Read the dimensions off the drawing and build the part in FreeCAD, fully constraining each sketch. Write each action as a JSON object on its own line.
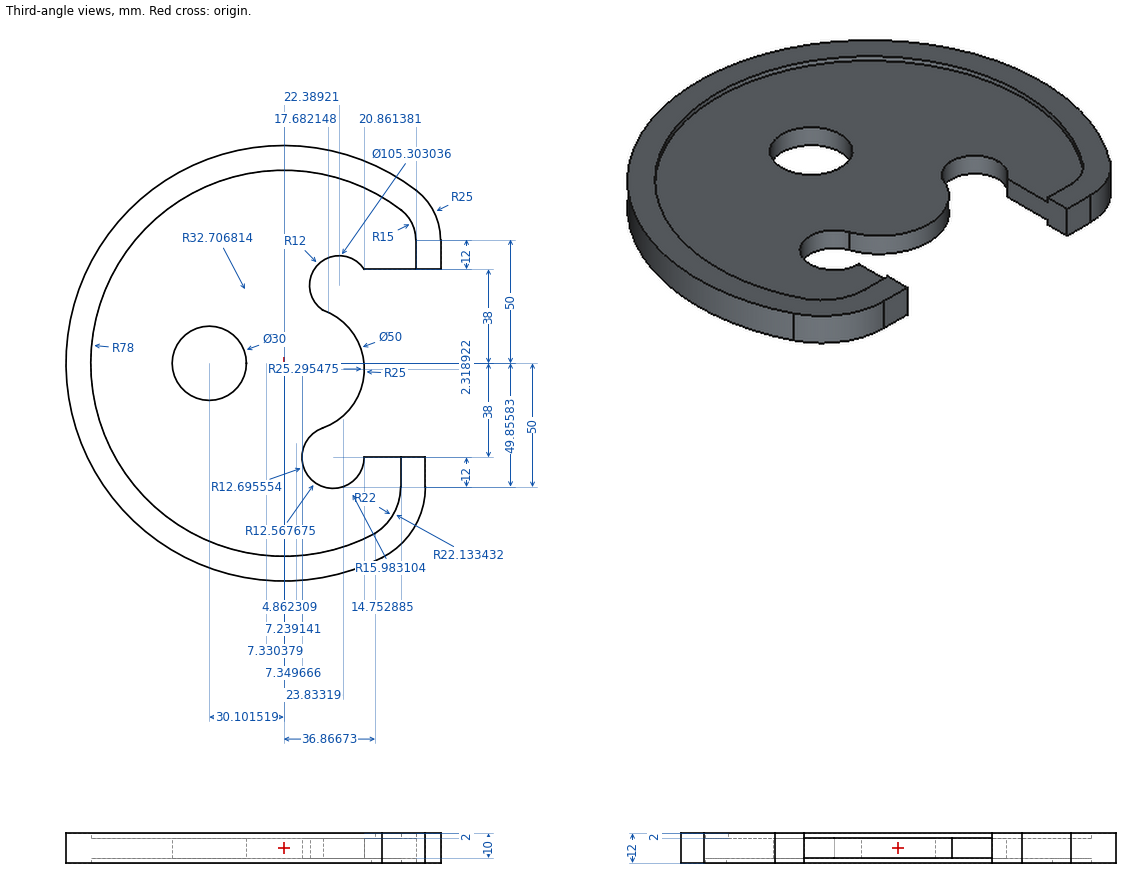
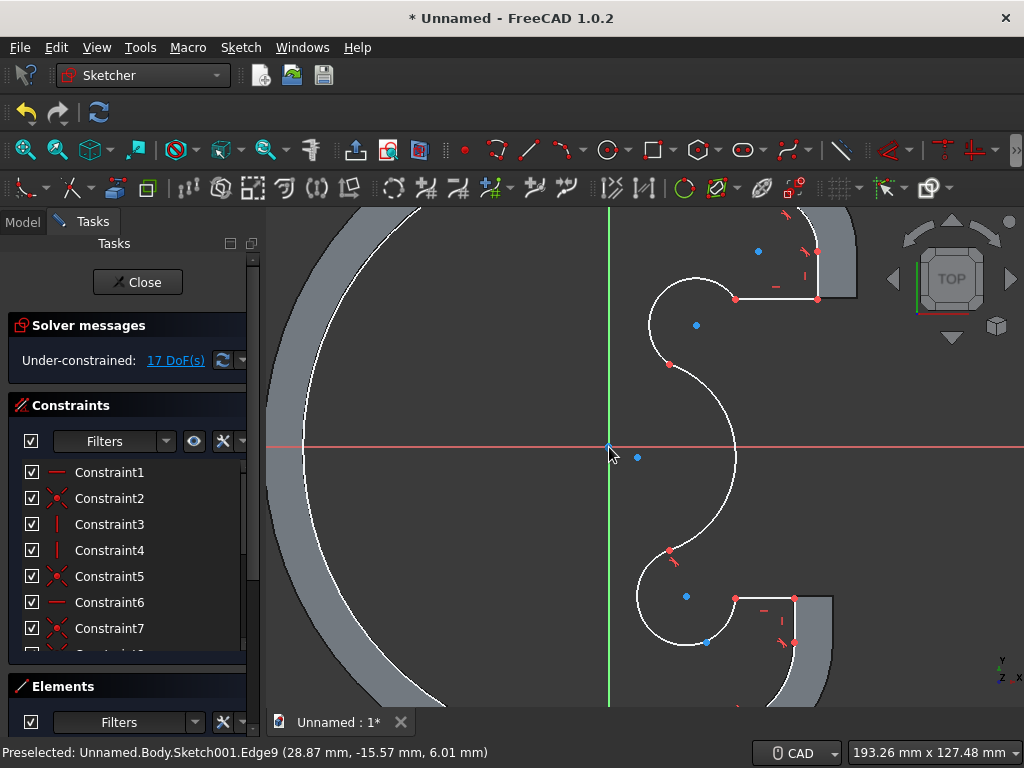
{"action": "left_click_drag", "start_coordinate": [599, 437], "coordinate": [619, 458]}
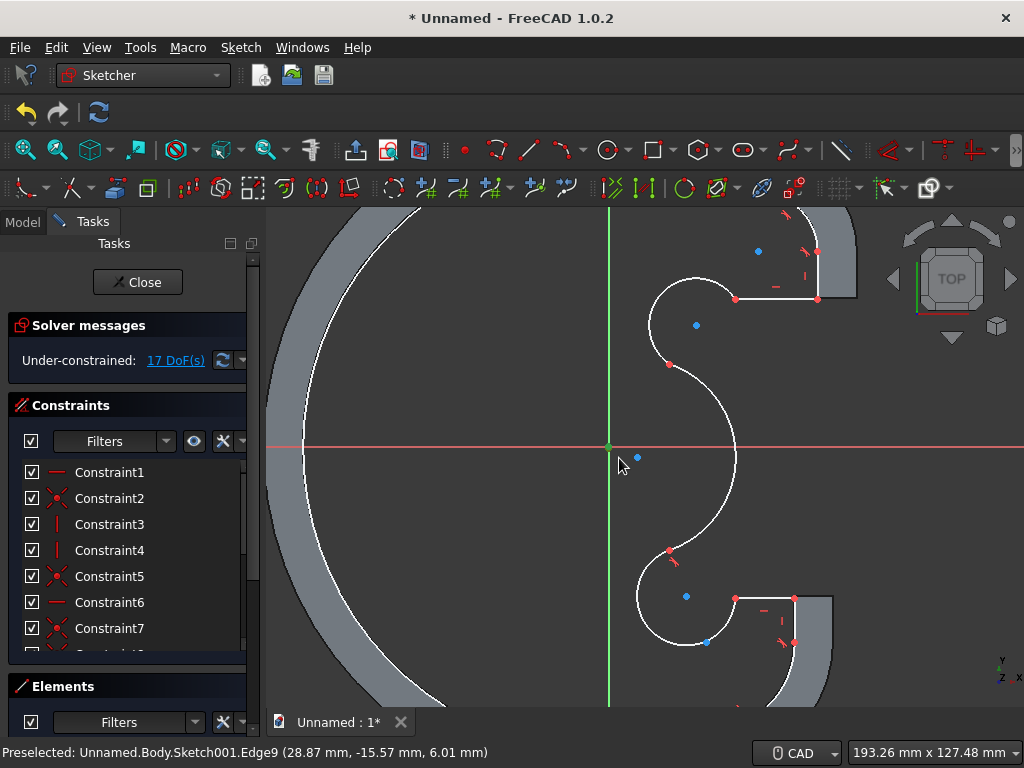
{"action": "left_click", "coordinate": [944, 150]}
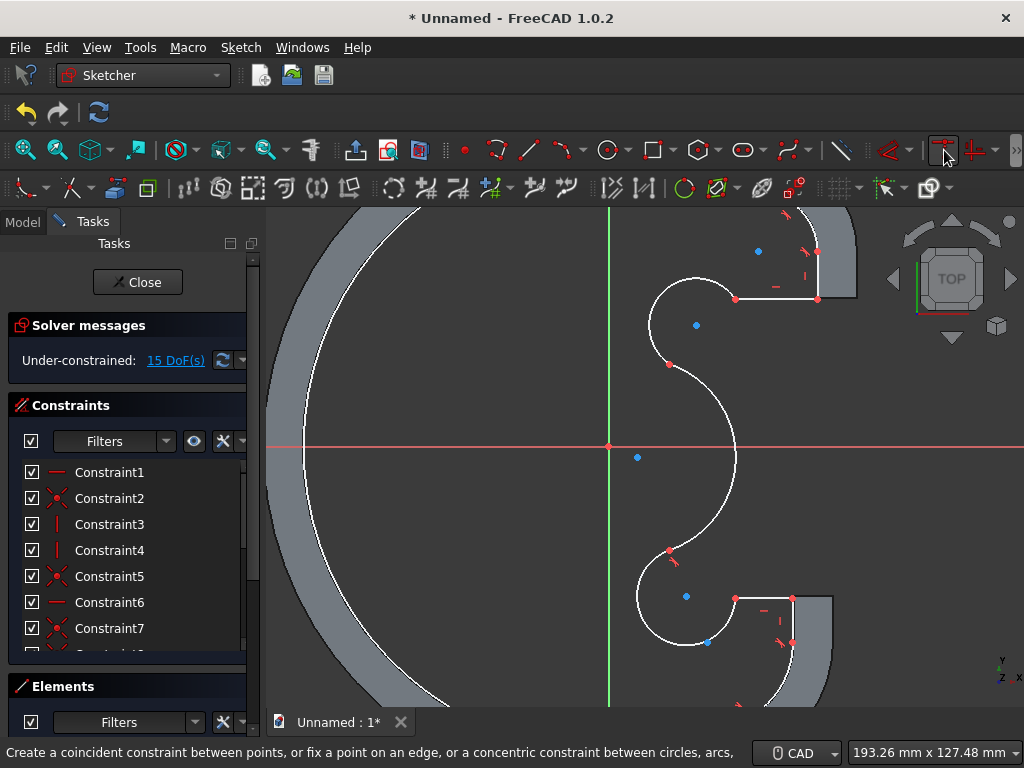
{"action": "left_click", "coordinate": [888, 150]}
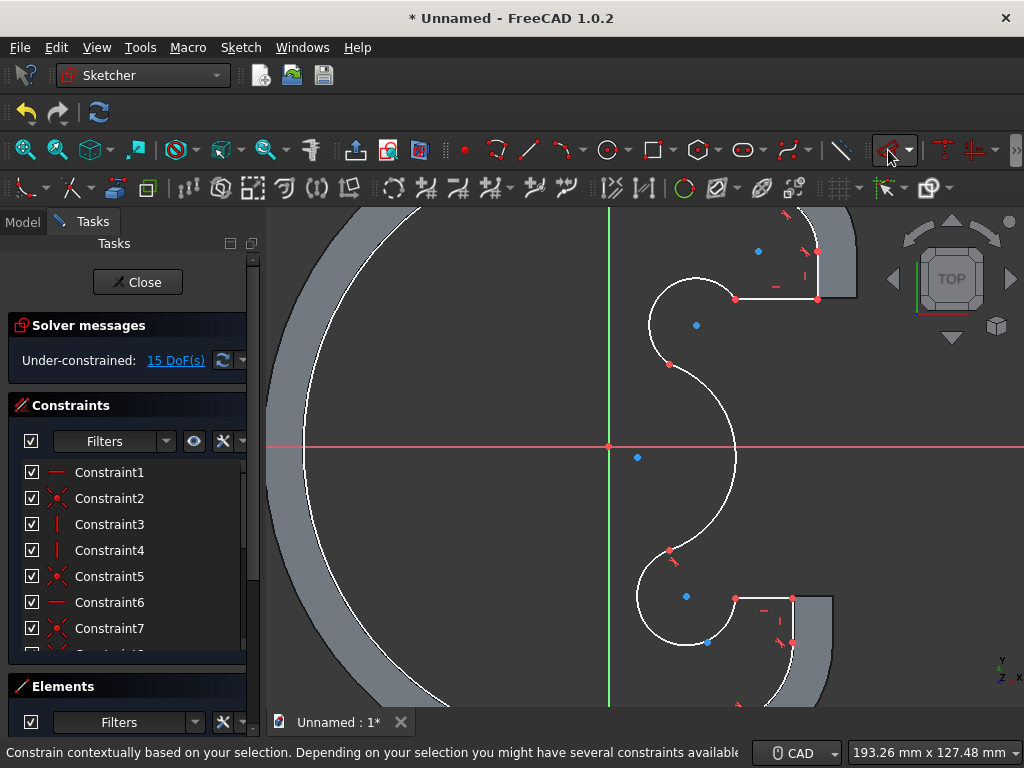
{"action": "left_click", "coordinate": [815, 236]}
{"action": "left_click", "coordinate": [847, 272]}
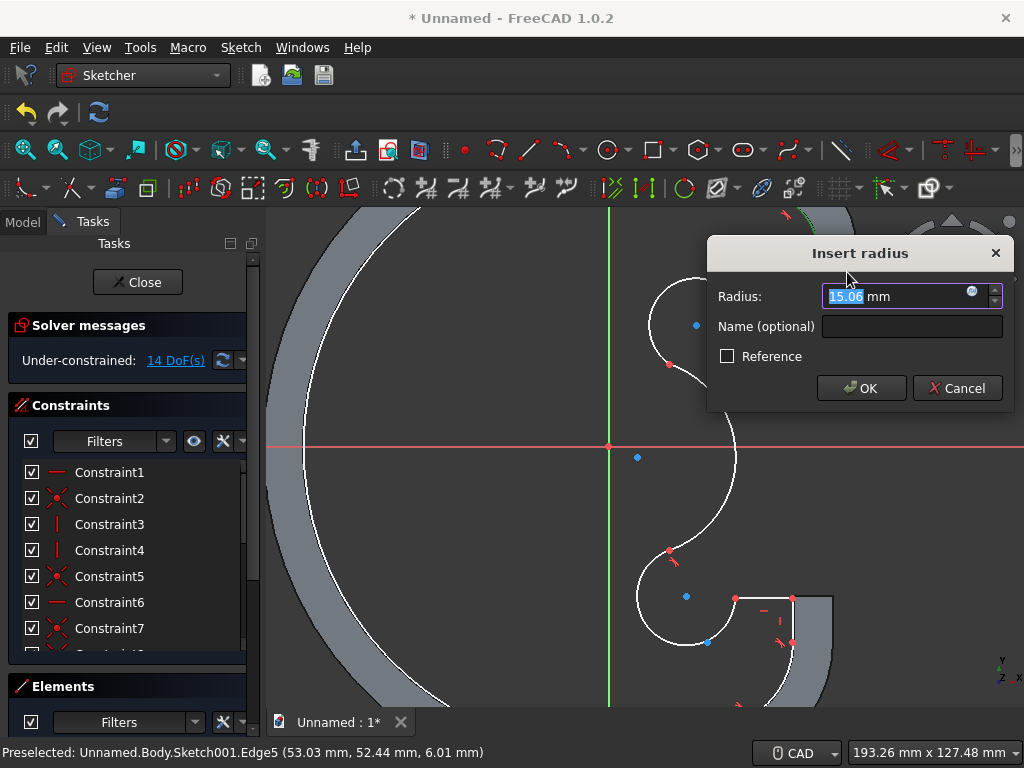
{"action": "type", "text": "15"}
{"action": "key", "text": "Return"}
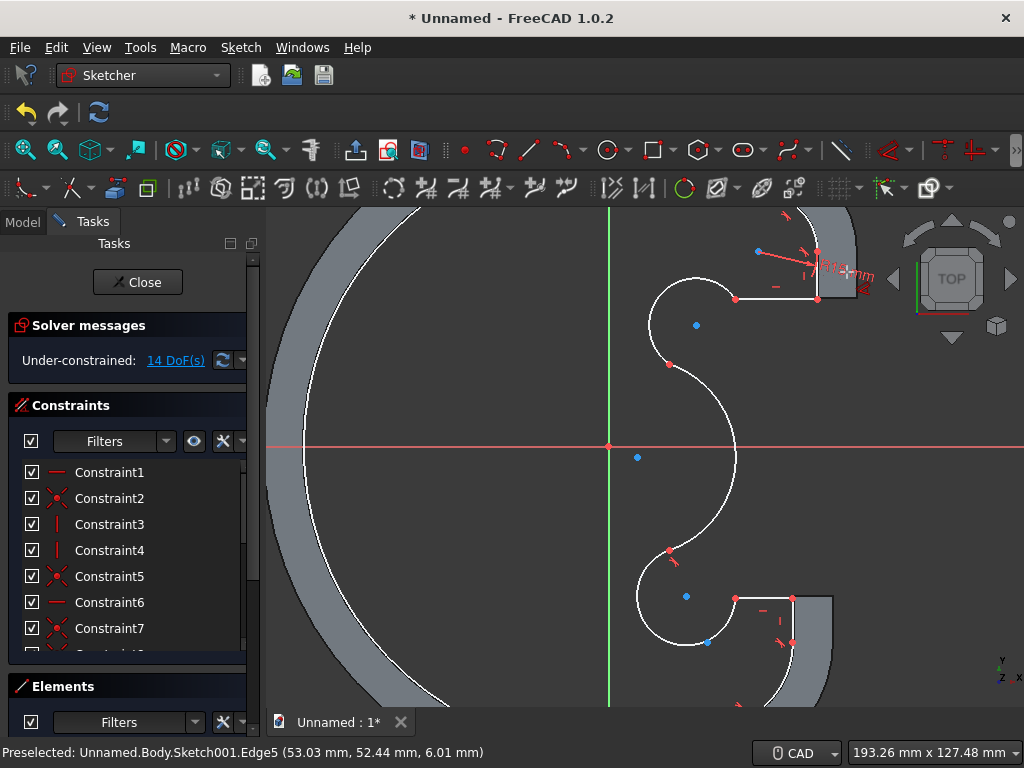
{"action": "left_click", "coordinate": [387, 657]}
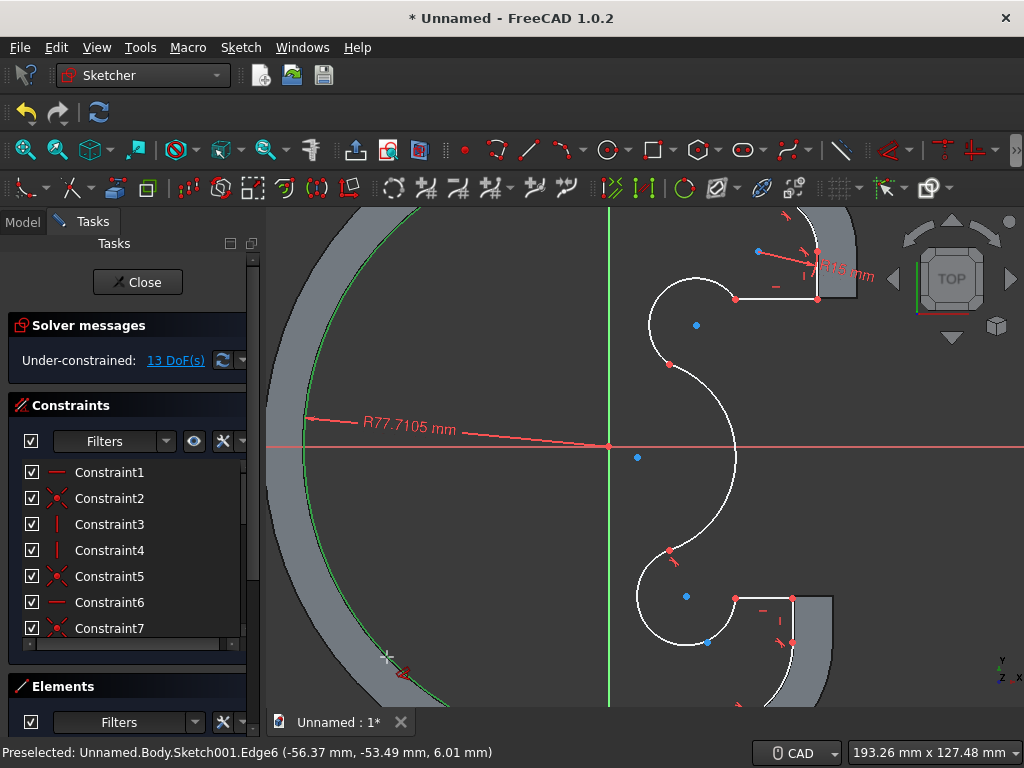
{"action": "key", "text": "Escape"}
{"action": "key", "text": "Escape"}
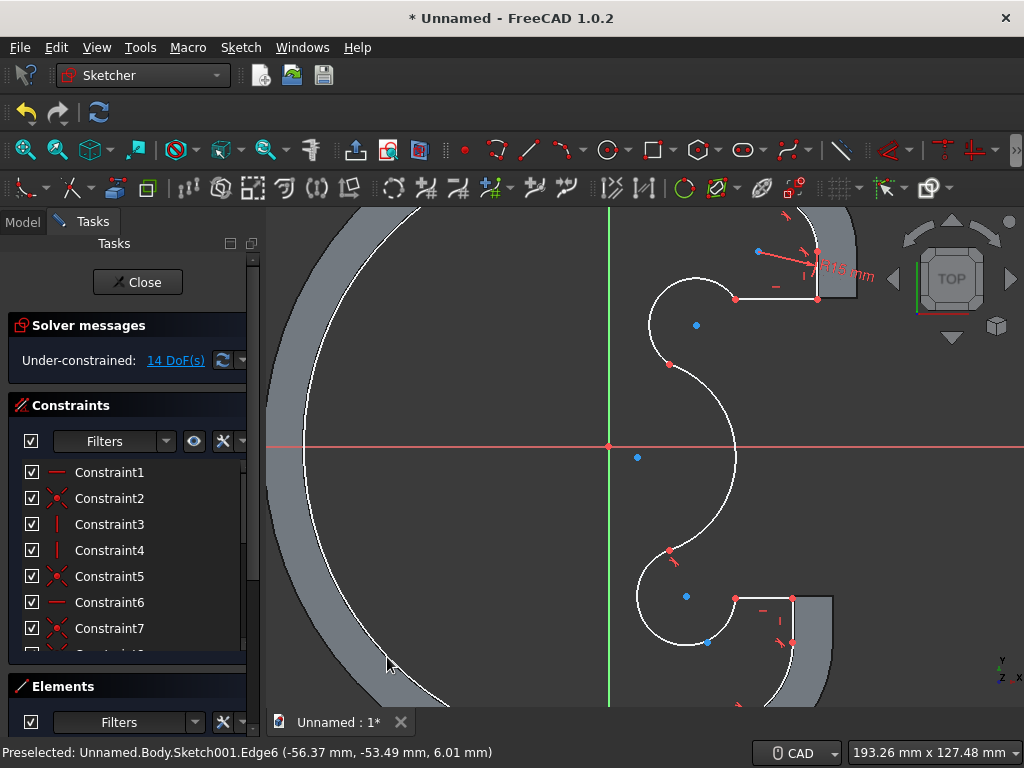
{"action": "left_click", "coordinate": [387, 657]}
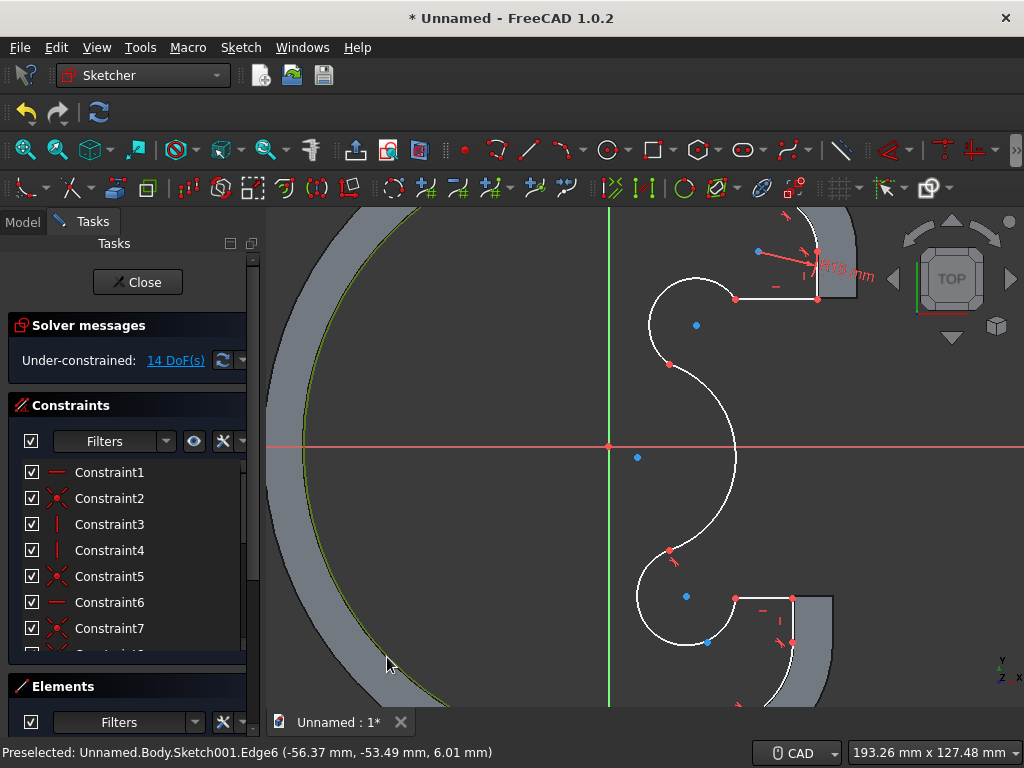
{"action": "key", "text": "k r"}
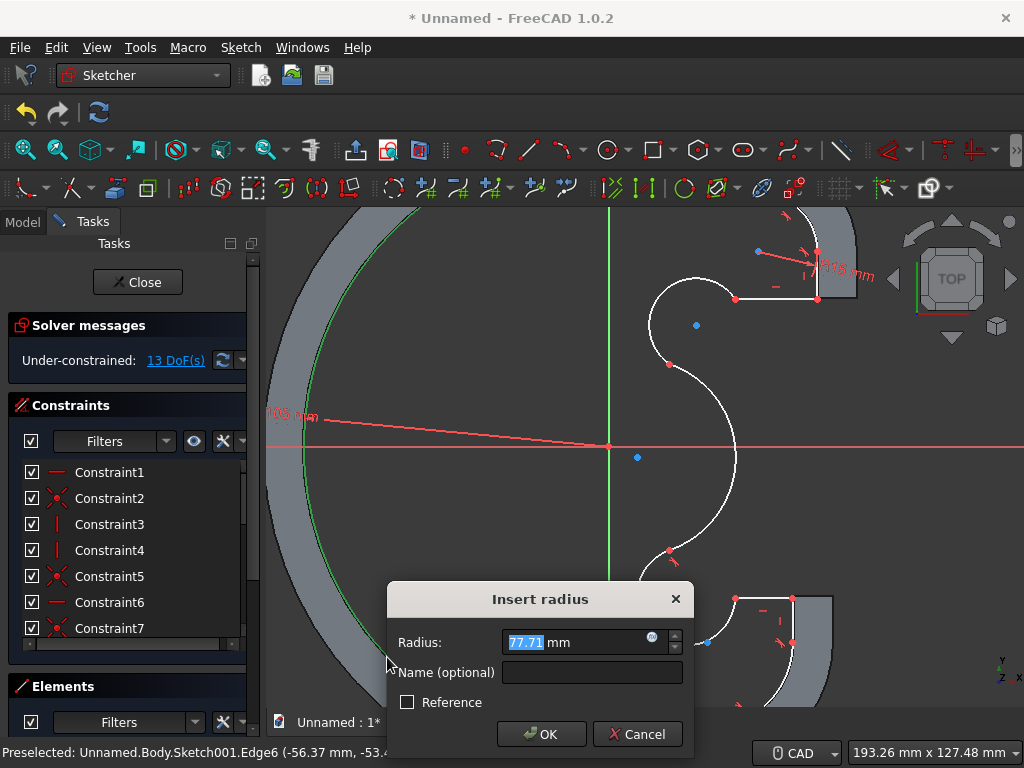
{"action": "type", "text": "78"}
{"action": "key", "text": "Return"}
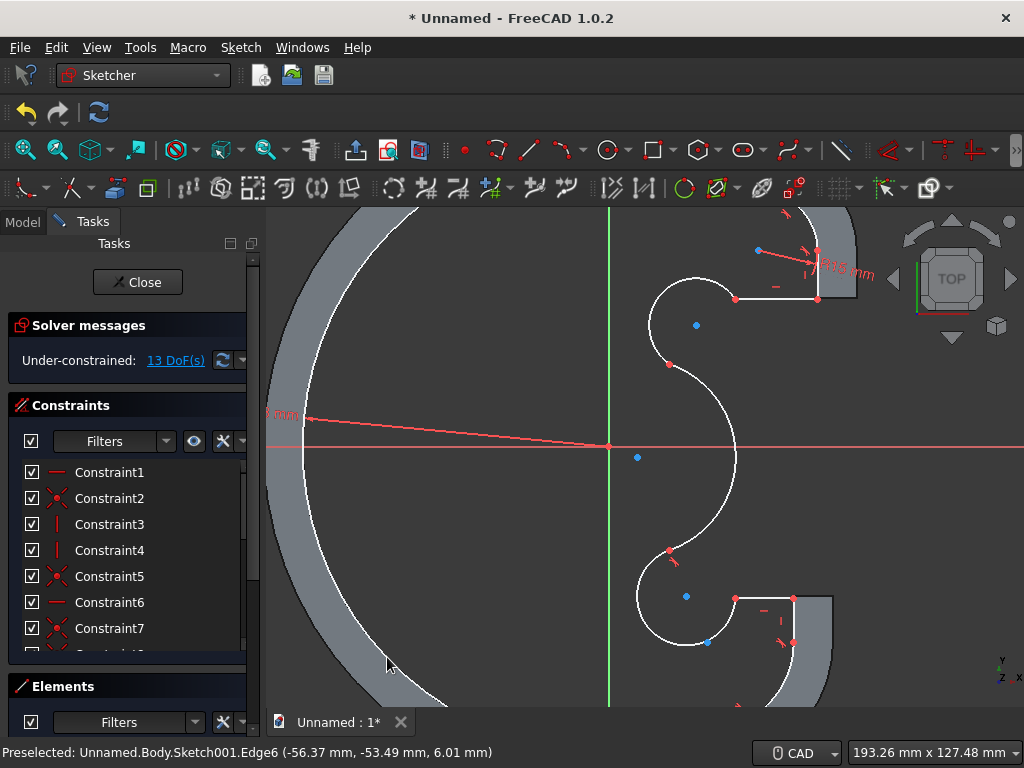
{"action": "left_click", "coordinate": [789, 671]}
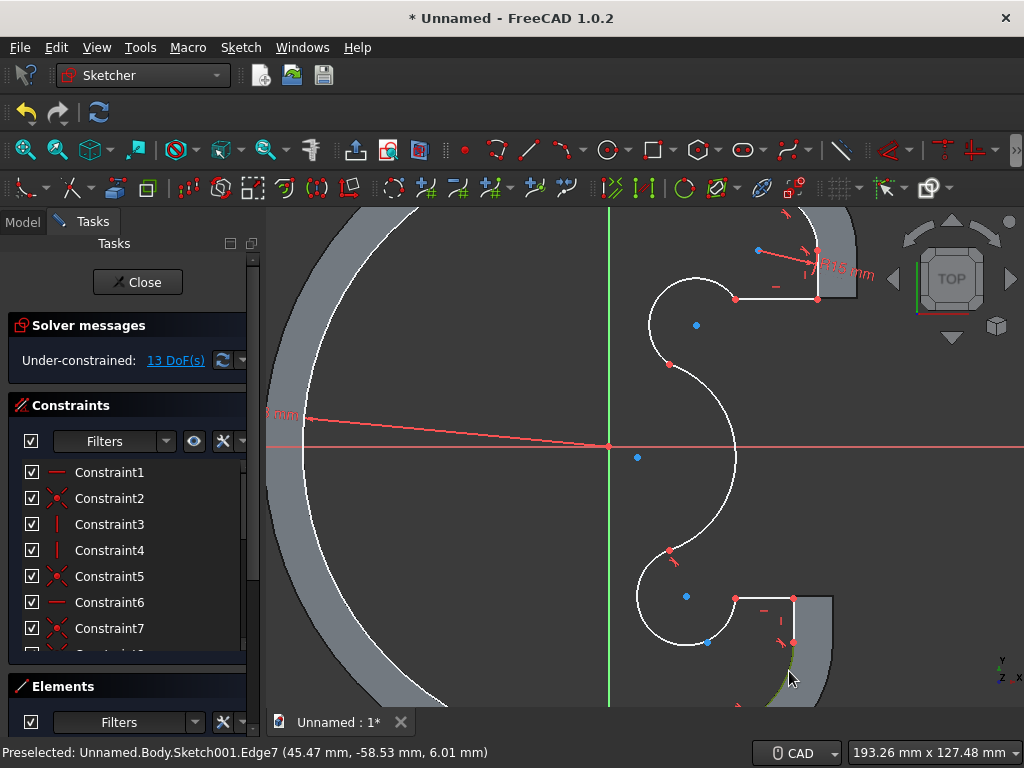
{"action": "key", "text": "k r"}